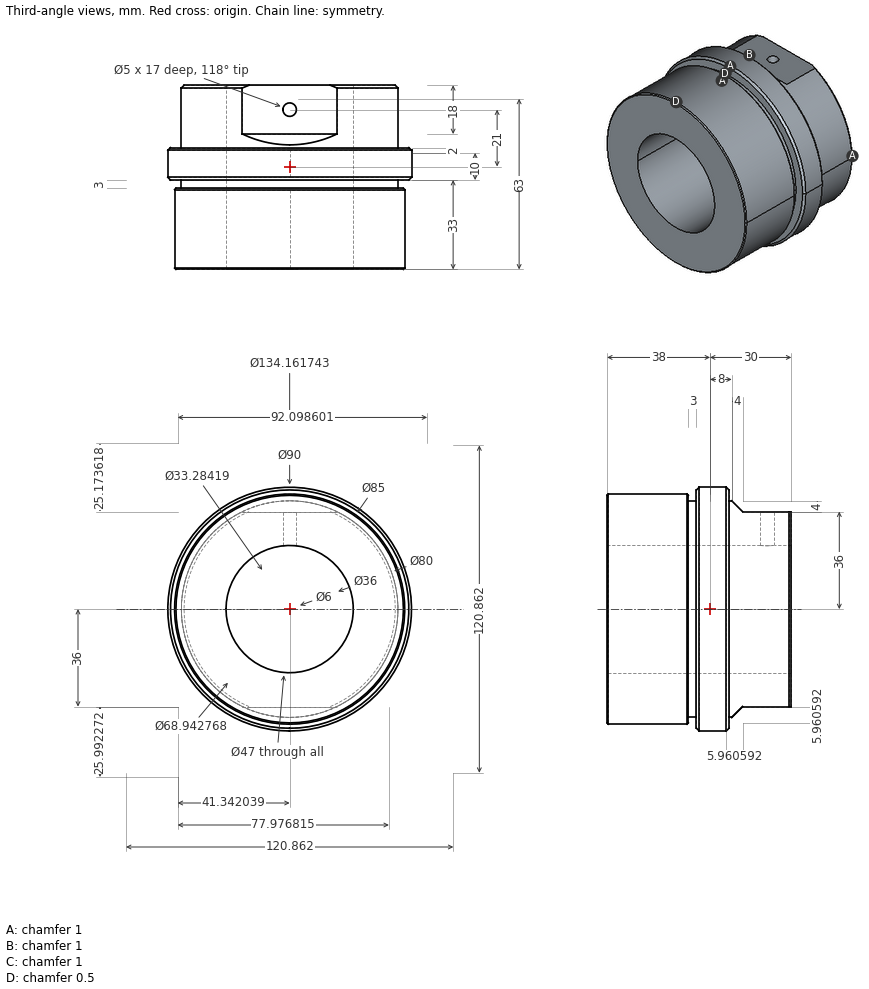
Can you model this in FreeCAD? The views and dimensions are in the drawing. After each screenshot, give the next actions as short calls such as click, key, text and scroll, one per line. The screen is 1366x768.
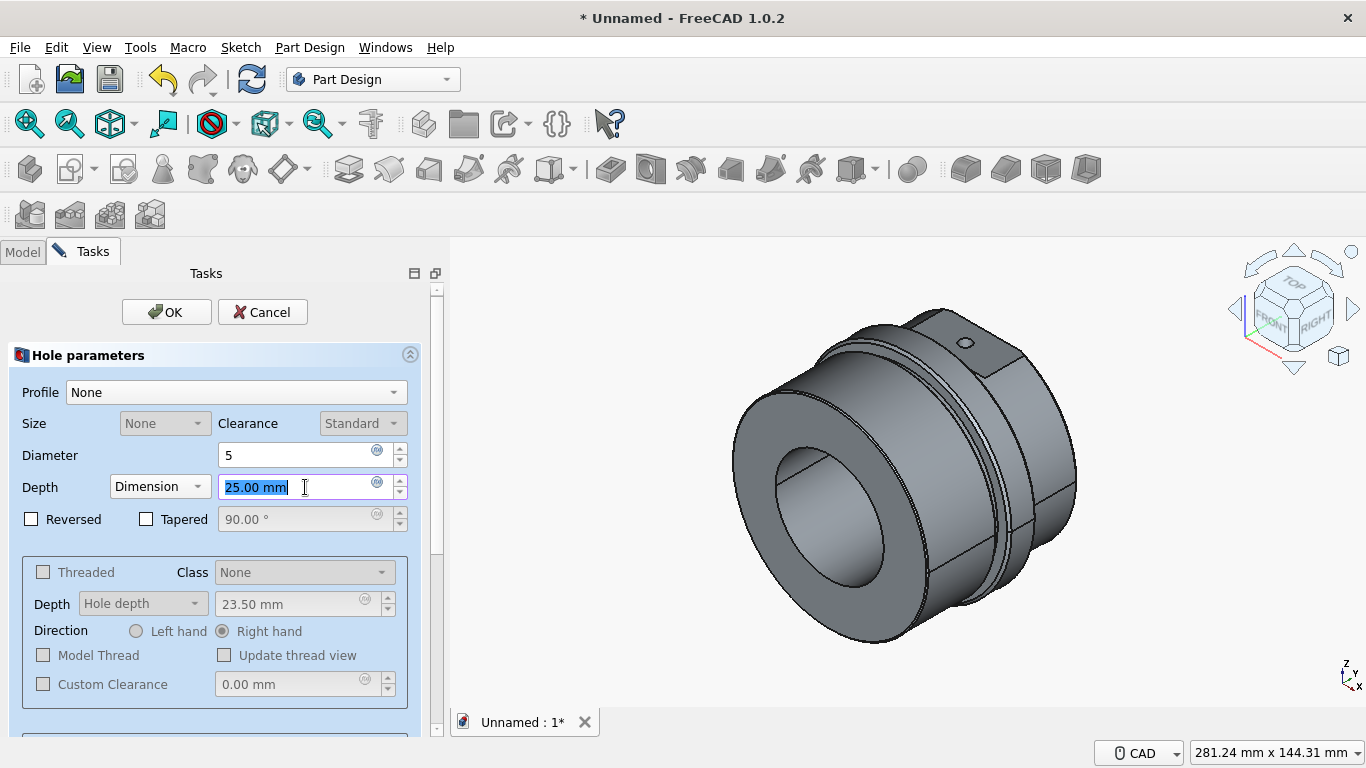
text(17)
key(Tab)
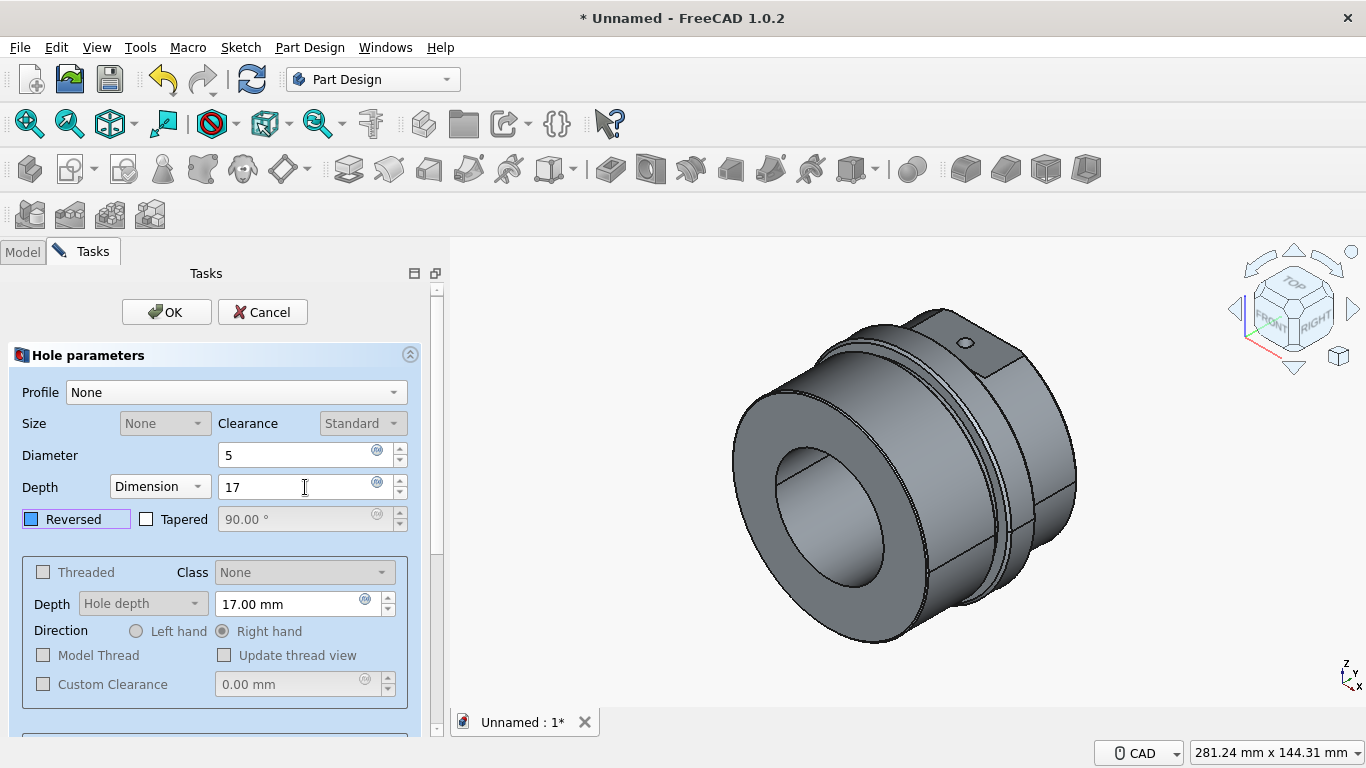
click(167, 312)